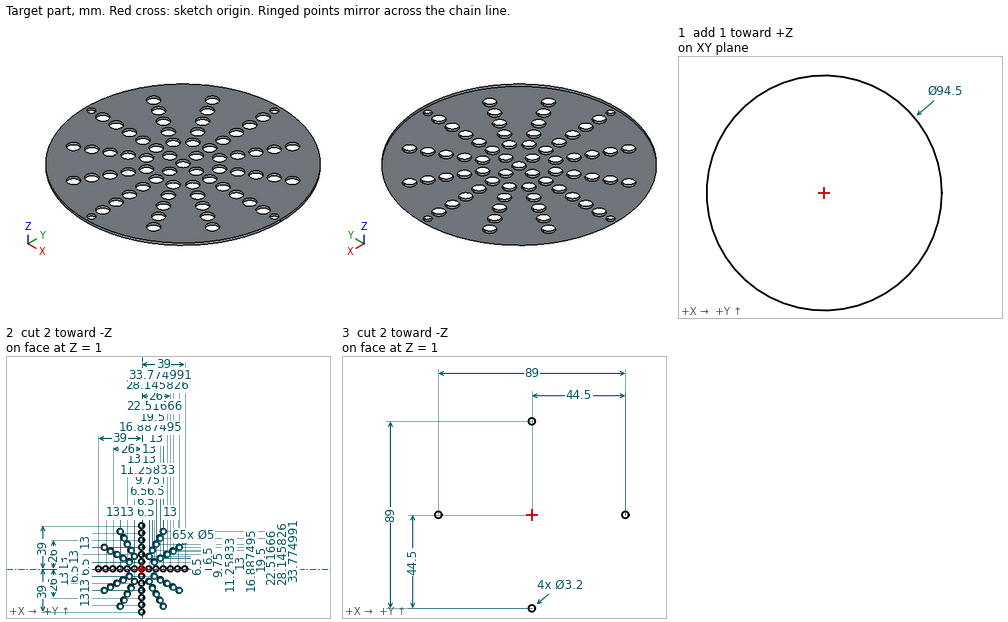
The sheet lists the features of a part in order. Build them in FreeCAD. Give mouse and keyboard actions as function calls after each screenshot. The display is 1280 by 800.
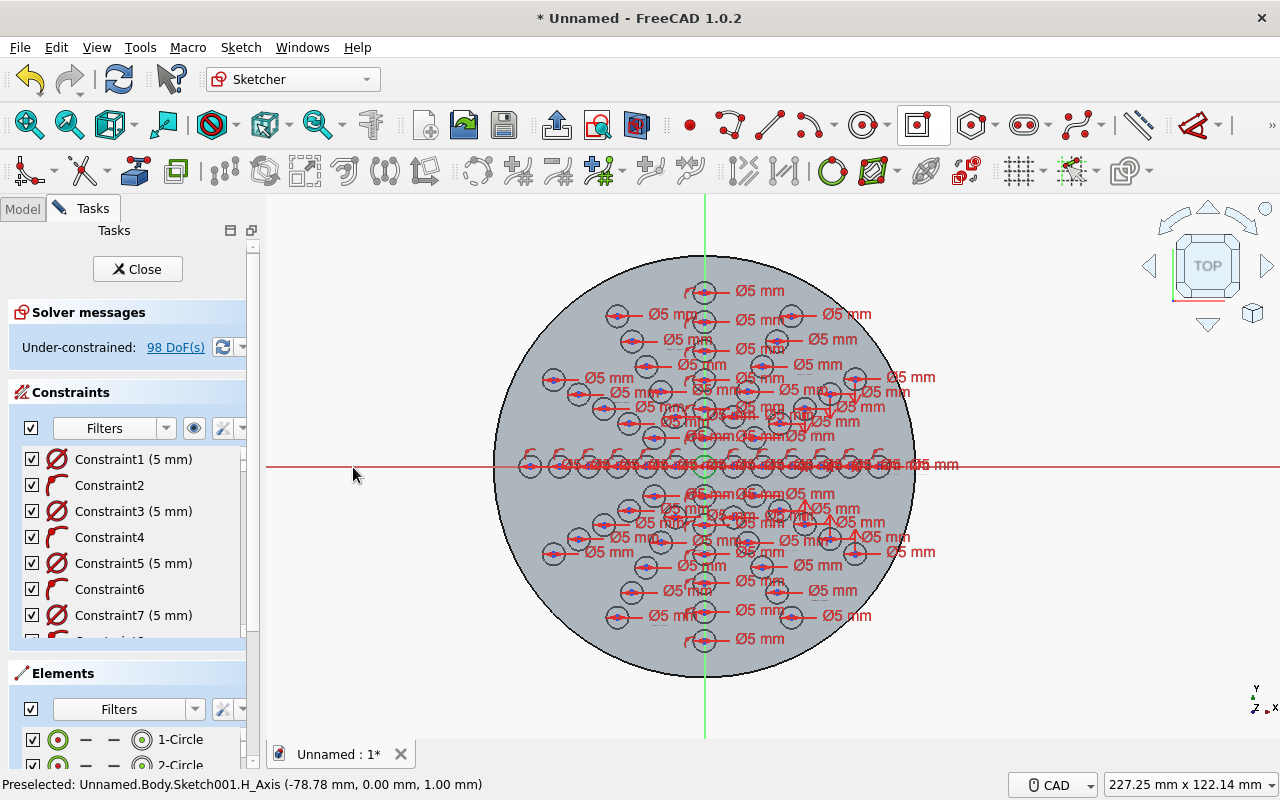
click(780, 424)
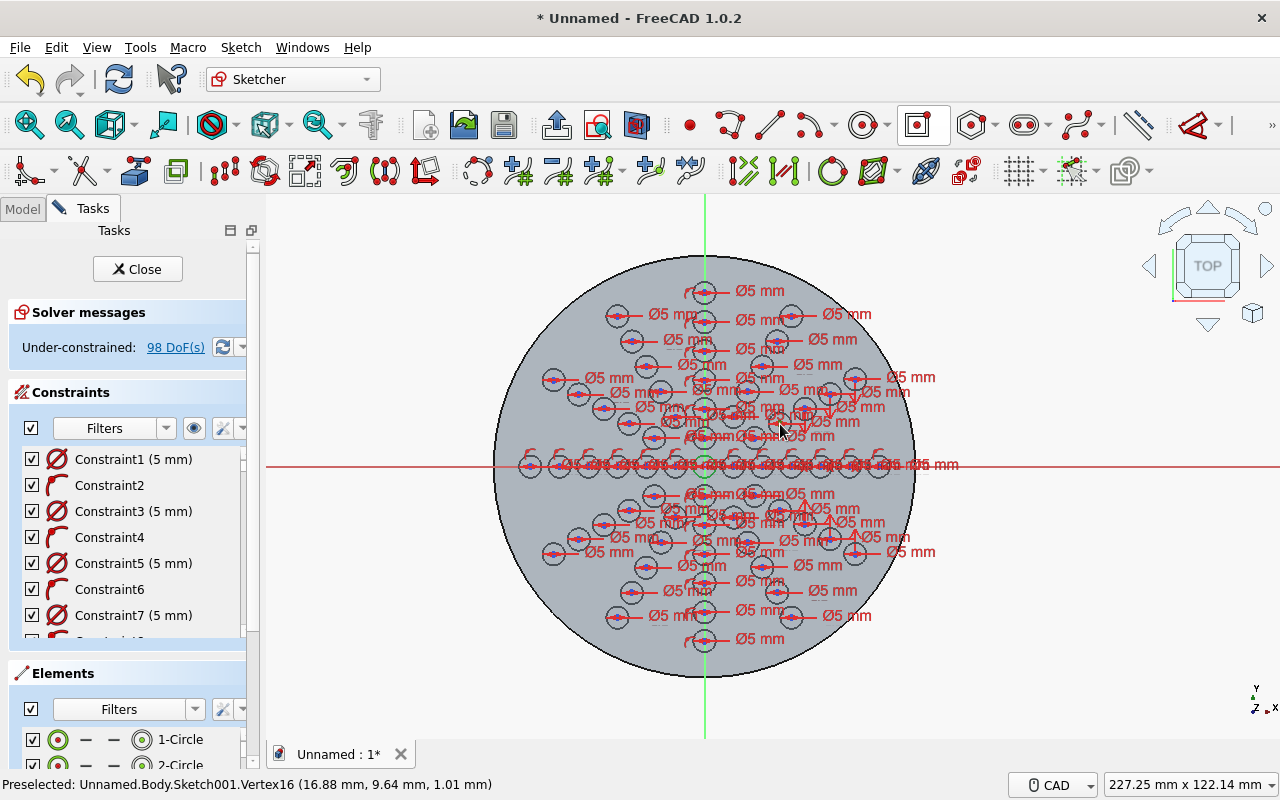
click(780, 511)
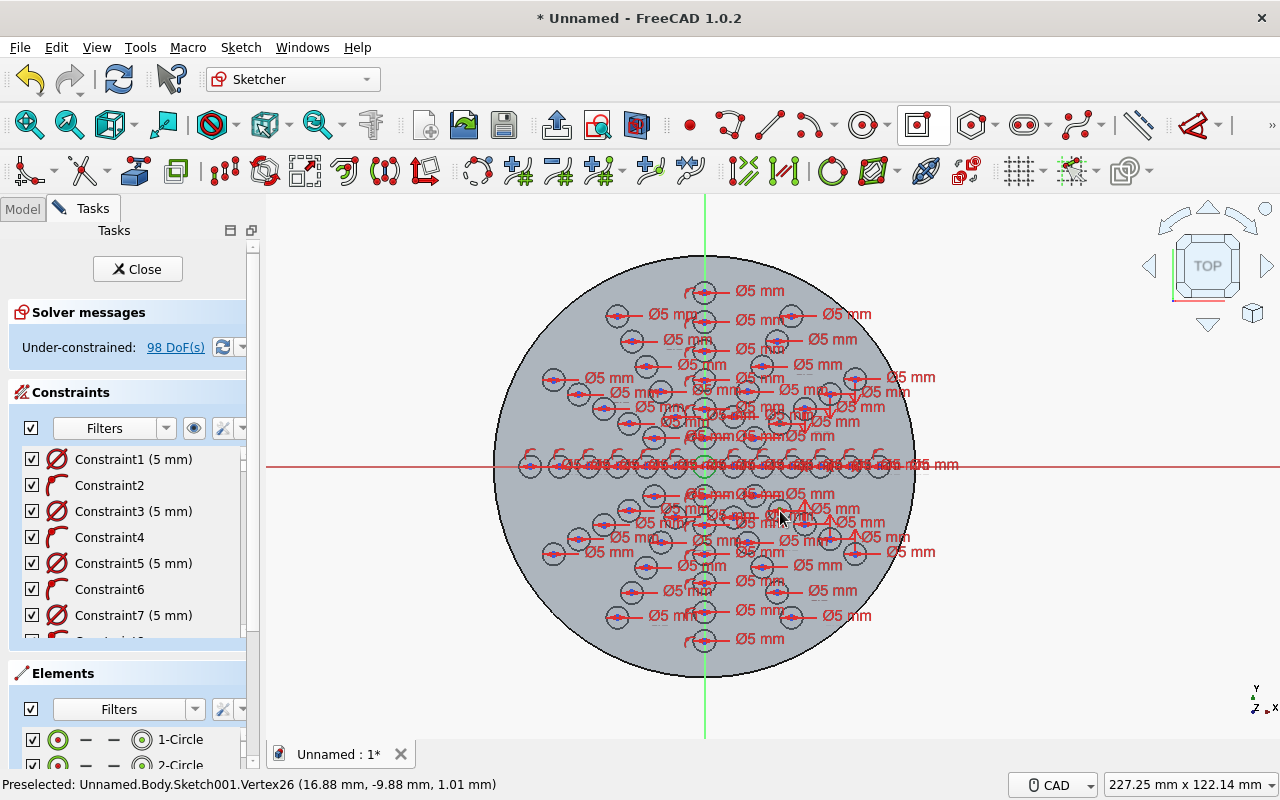
click(353, 467)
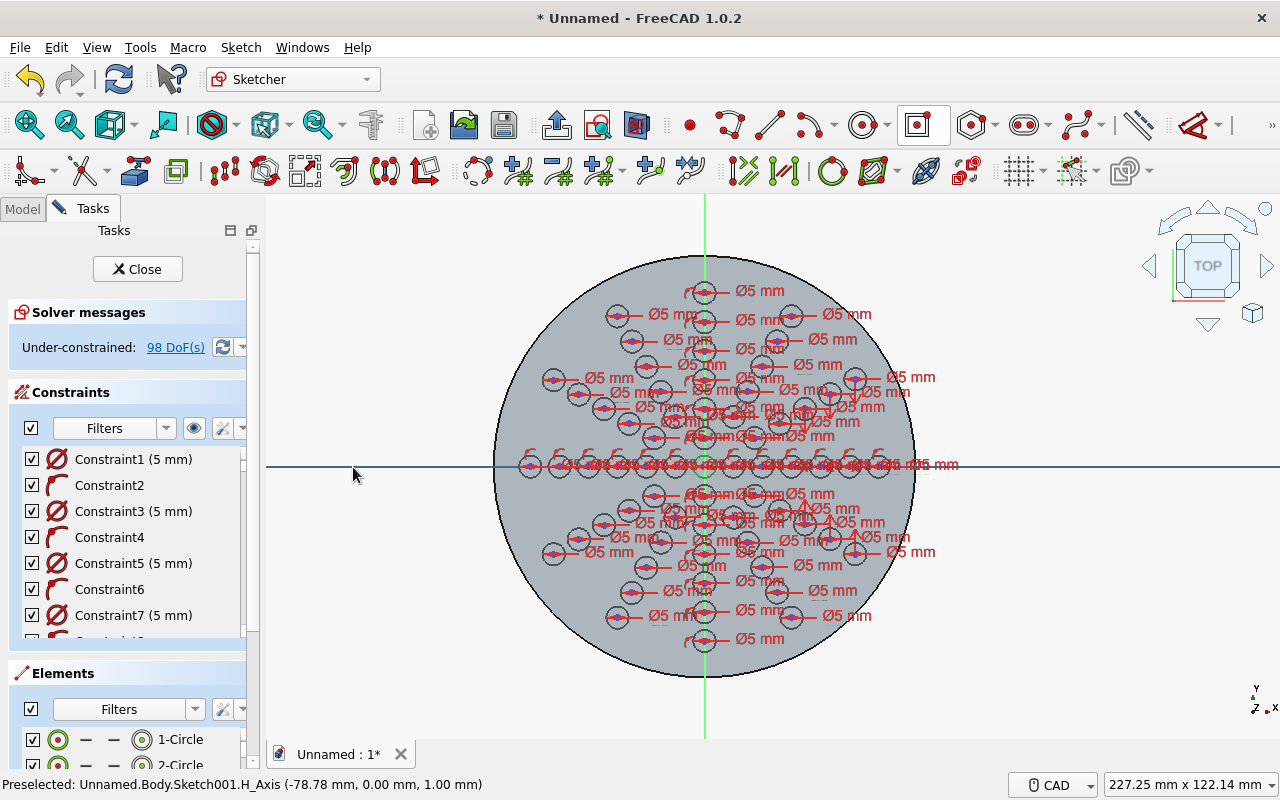
key(s)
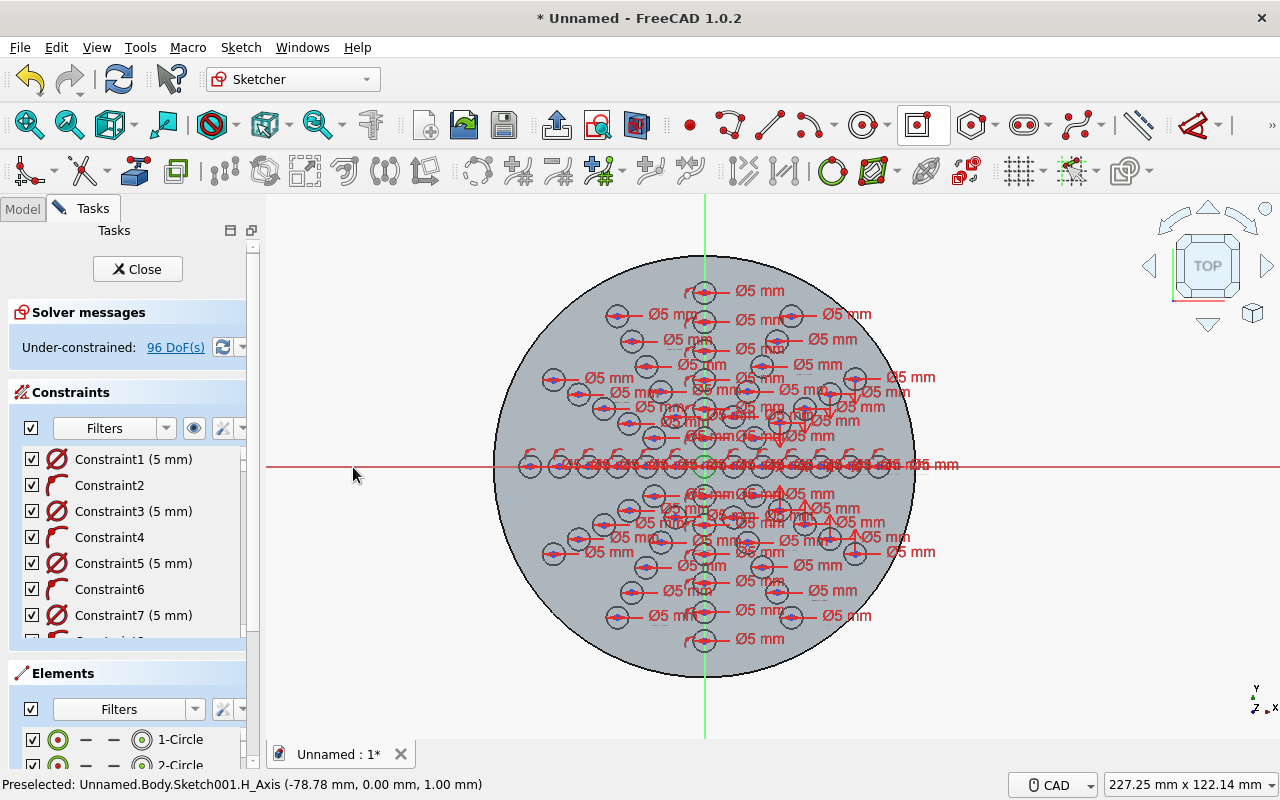
click(755, 438)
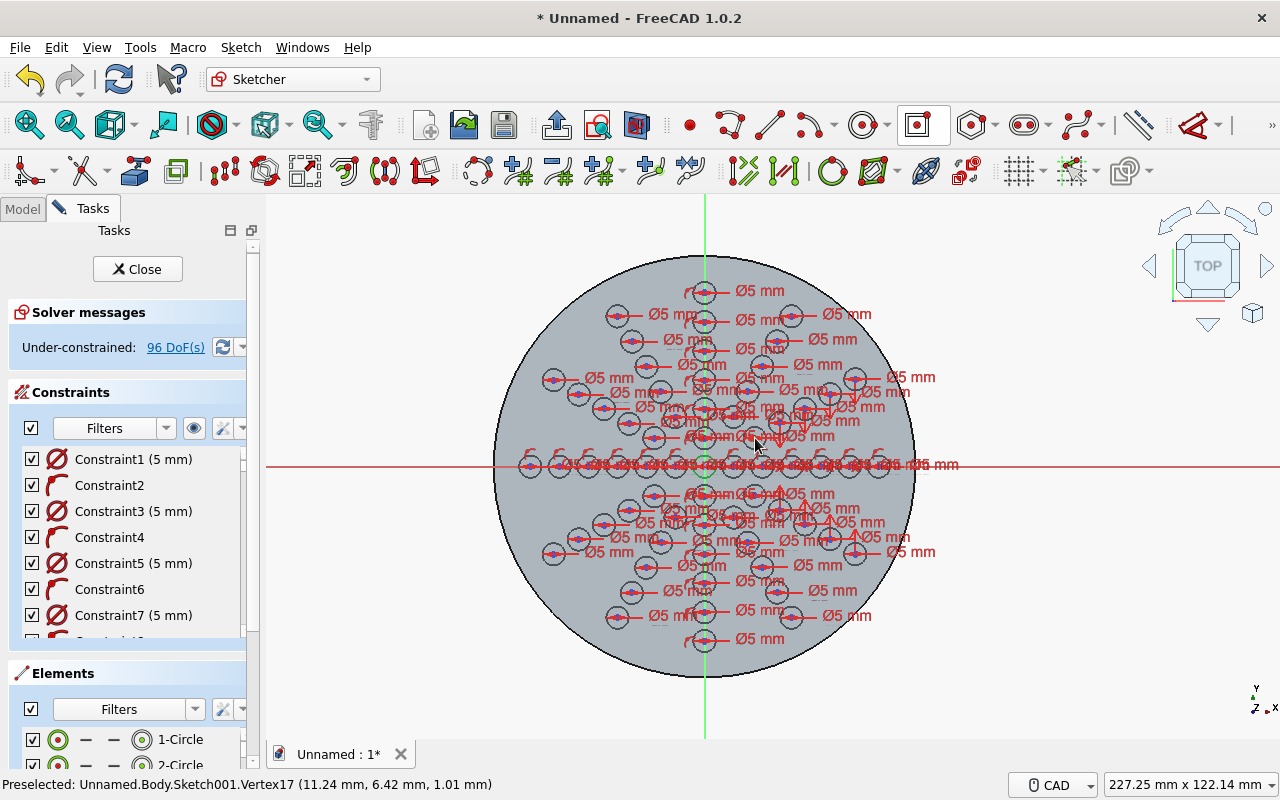
click(755, 496)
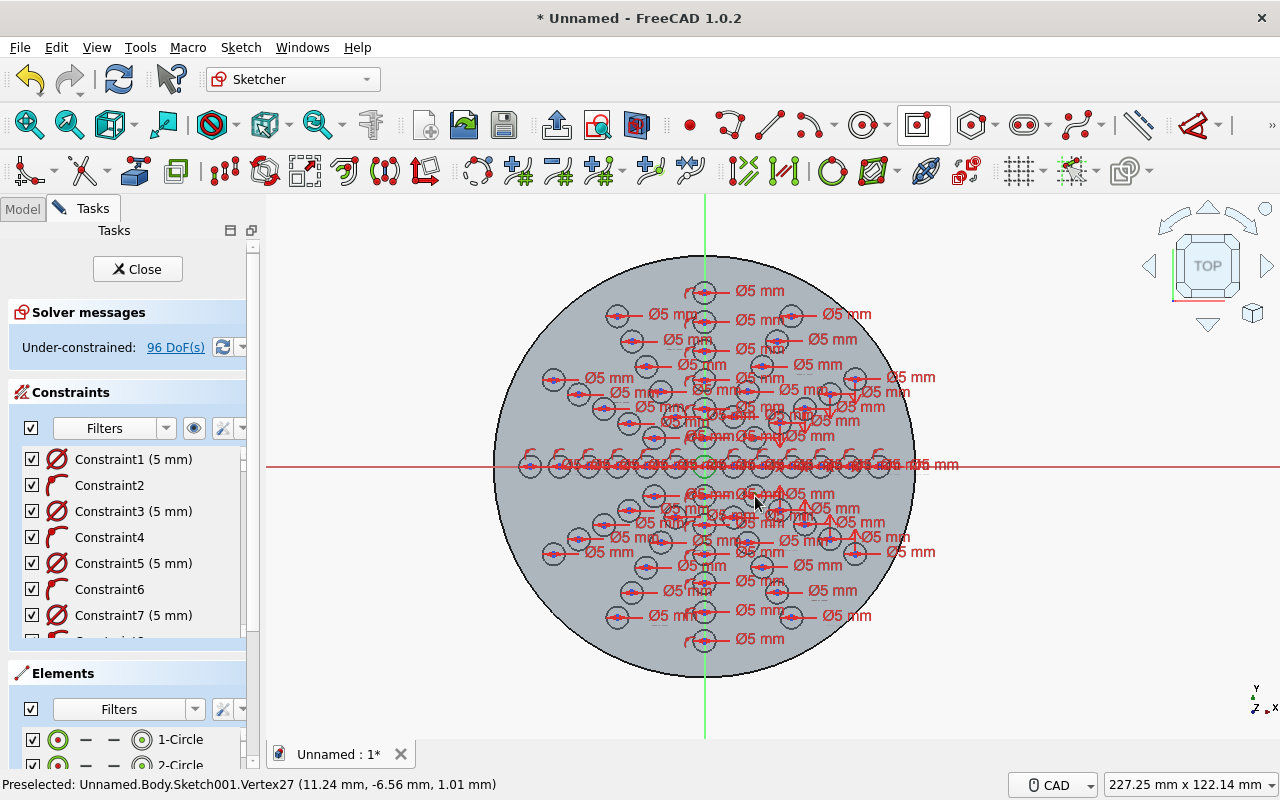
click(353, 467)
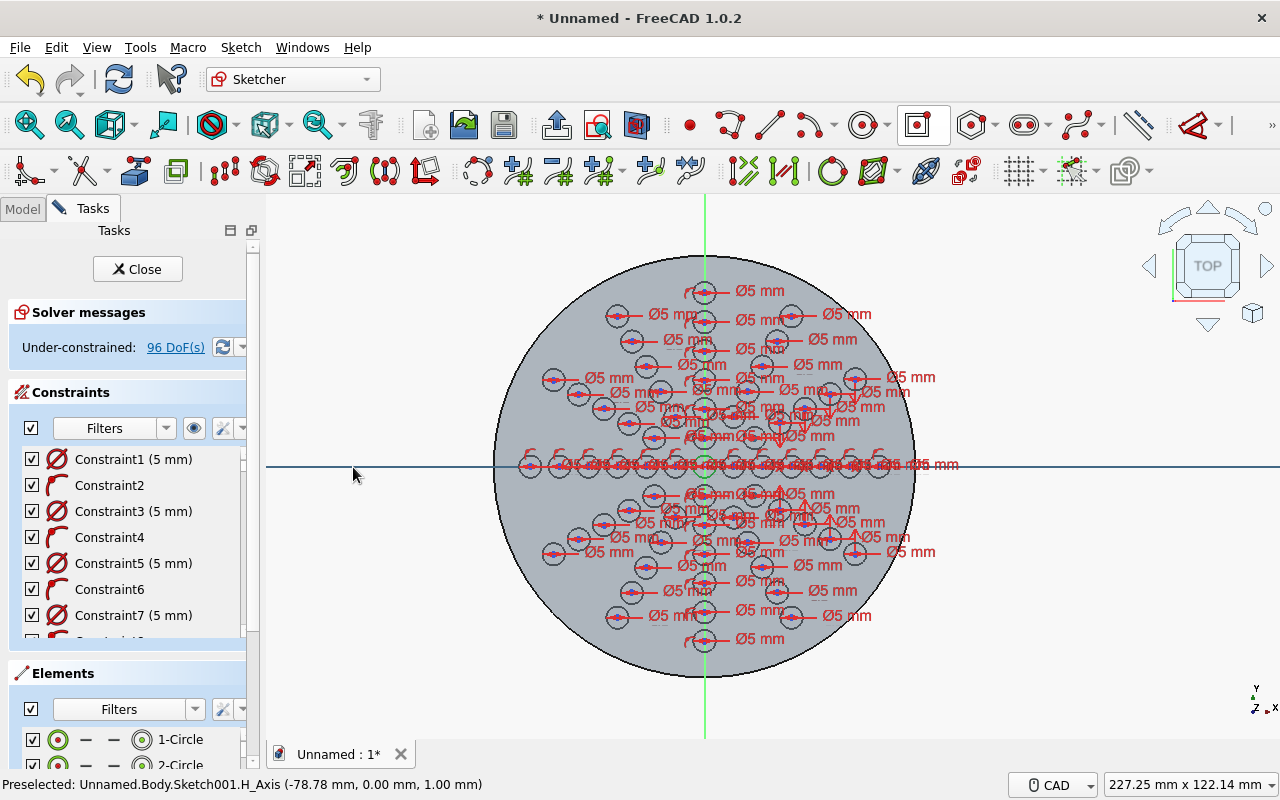
key(s)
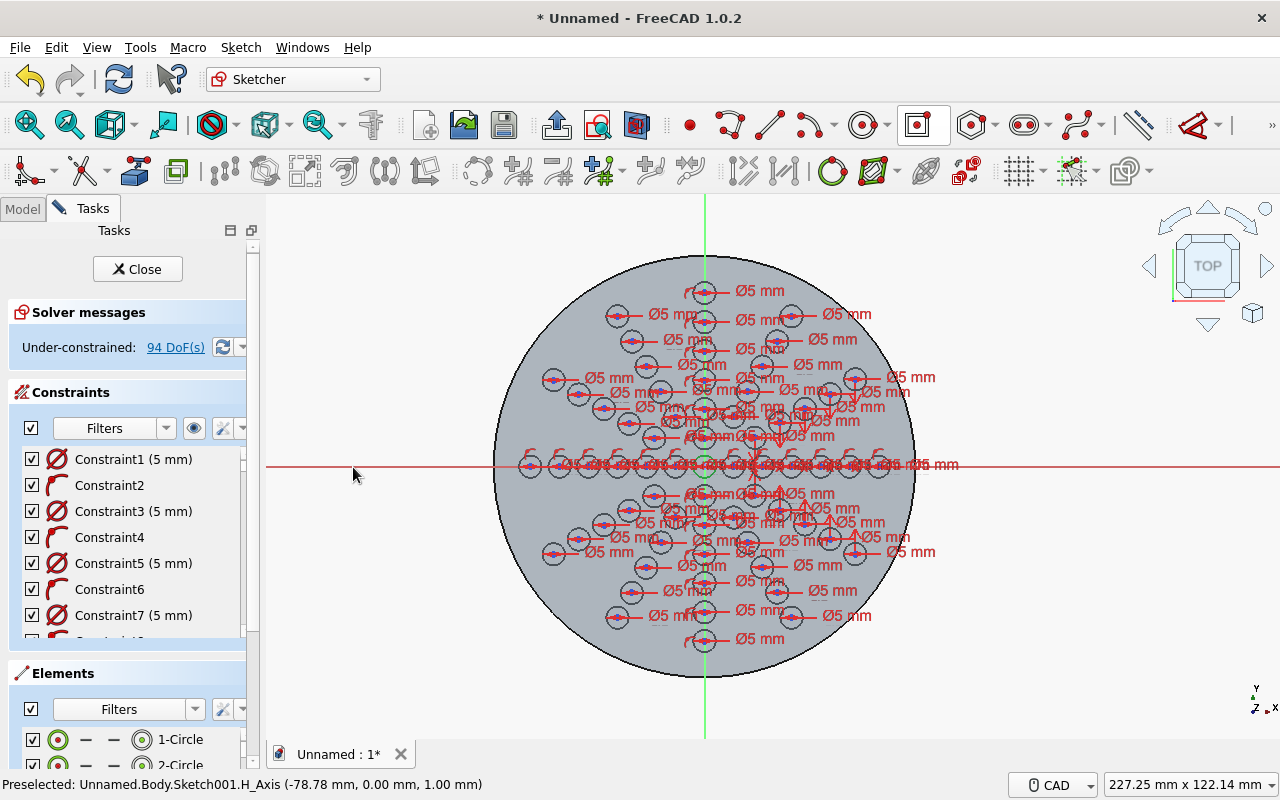
click(792, 316)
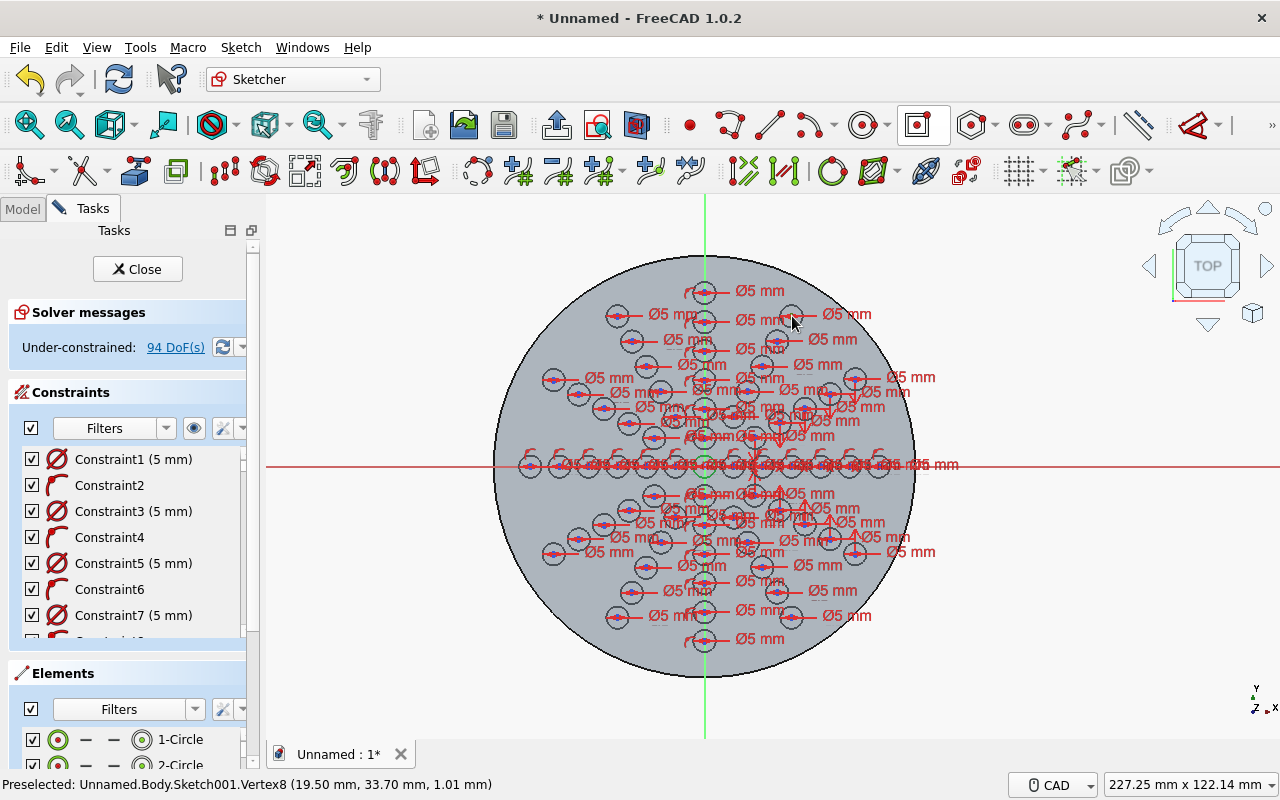
click(792, 618)